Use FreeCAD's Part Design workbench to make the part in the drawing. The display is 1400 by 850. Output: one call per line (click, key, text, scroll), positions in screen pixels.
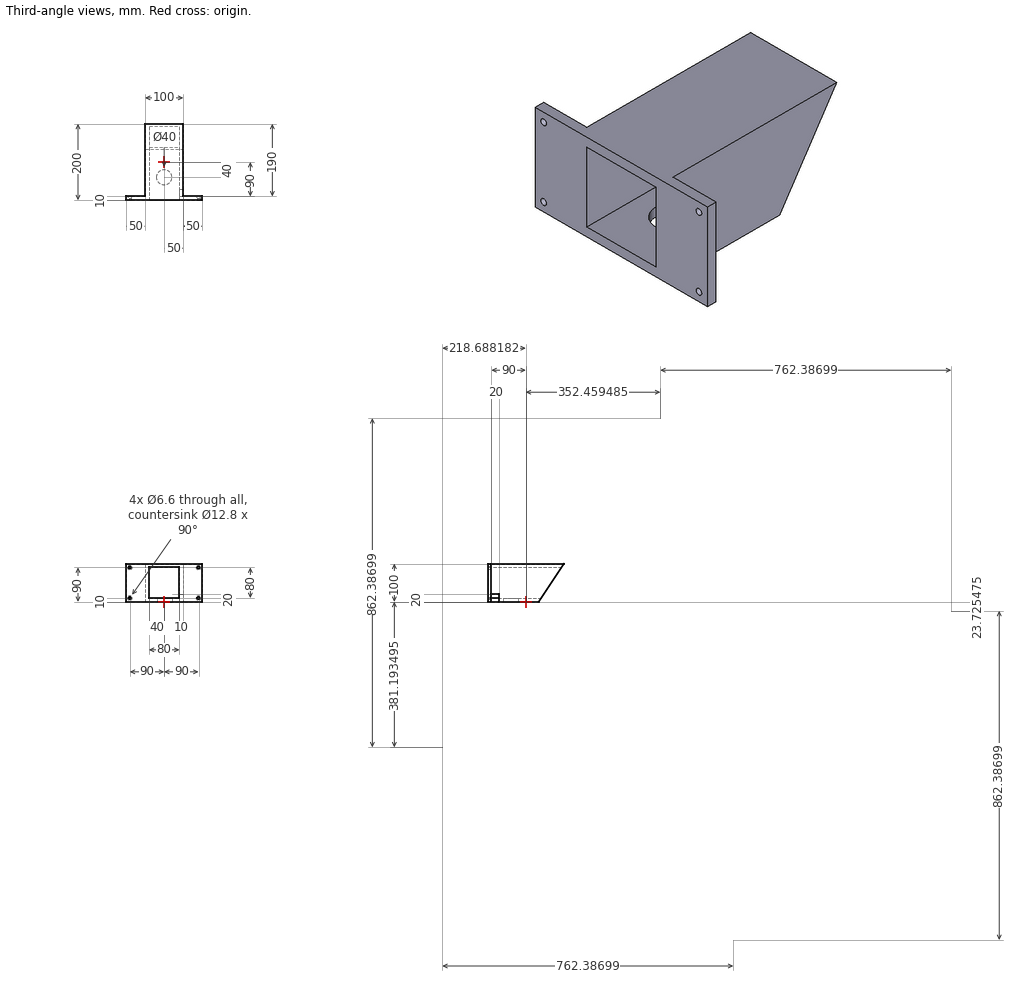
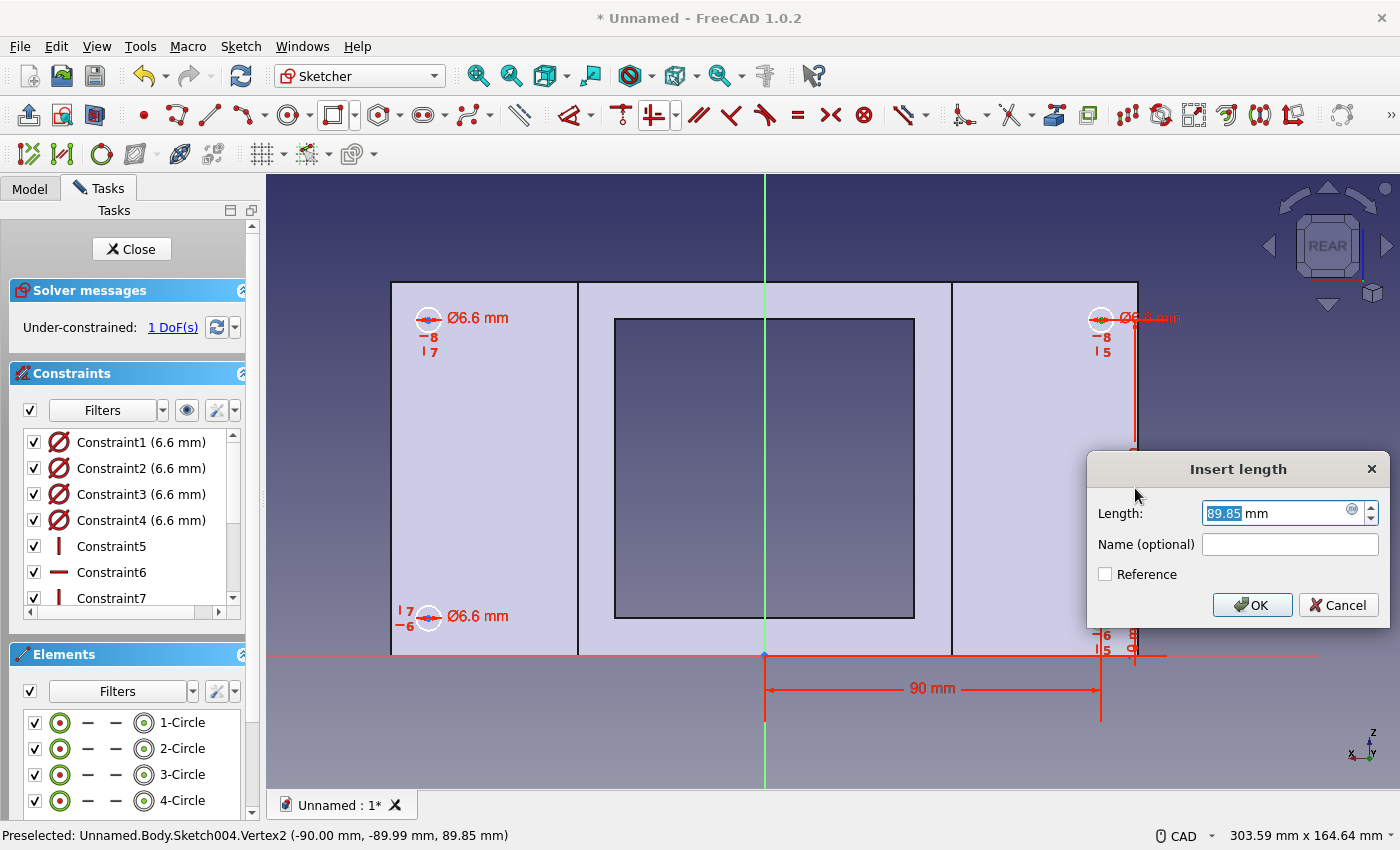
text(90)
key(Return)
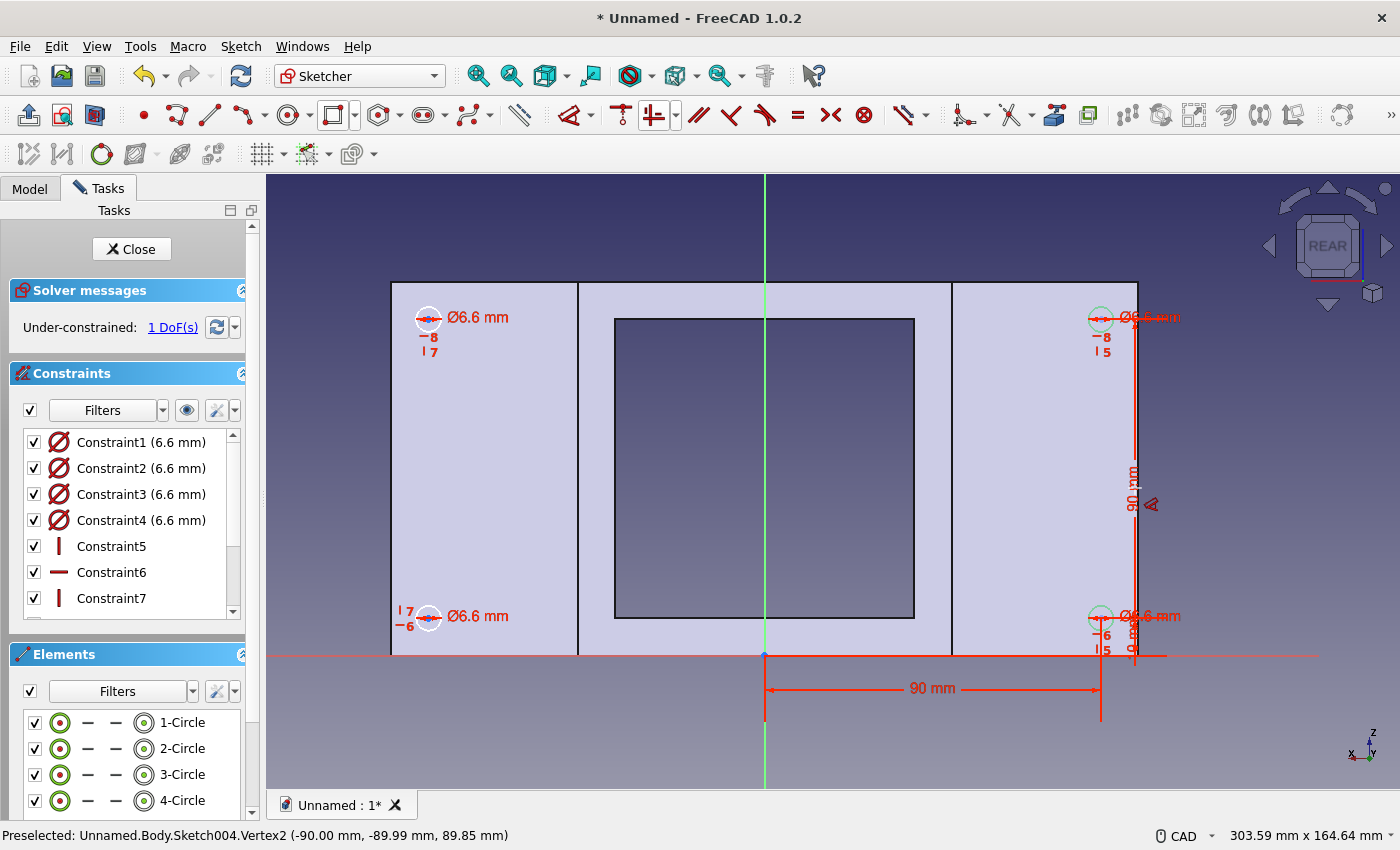
click(429, 618)
click(597, 690)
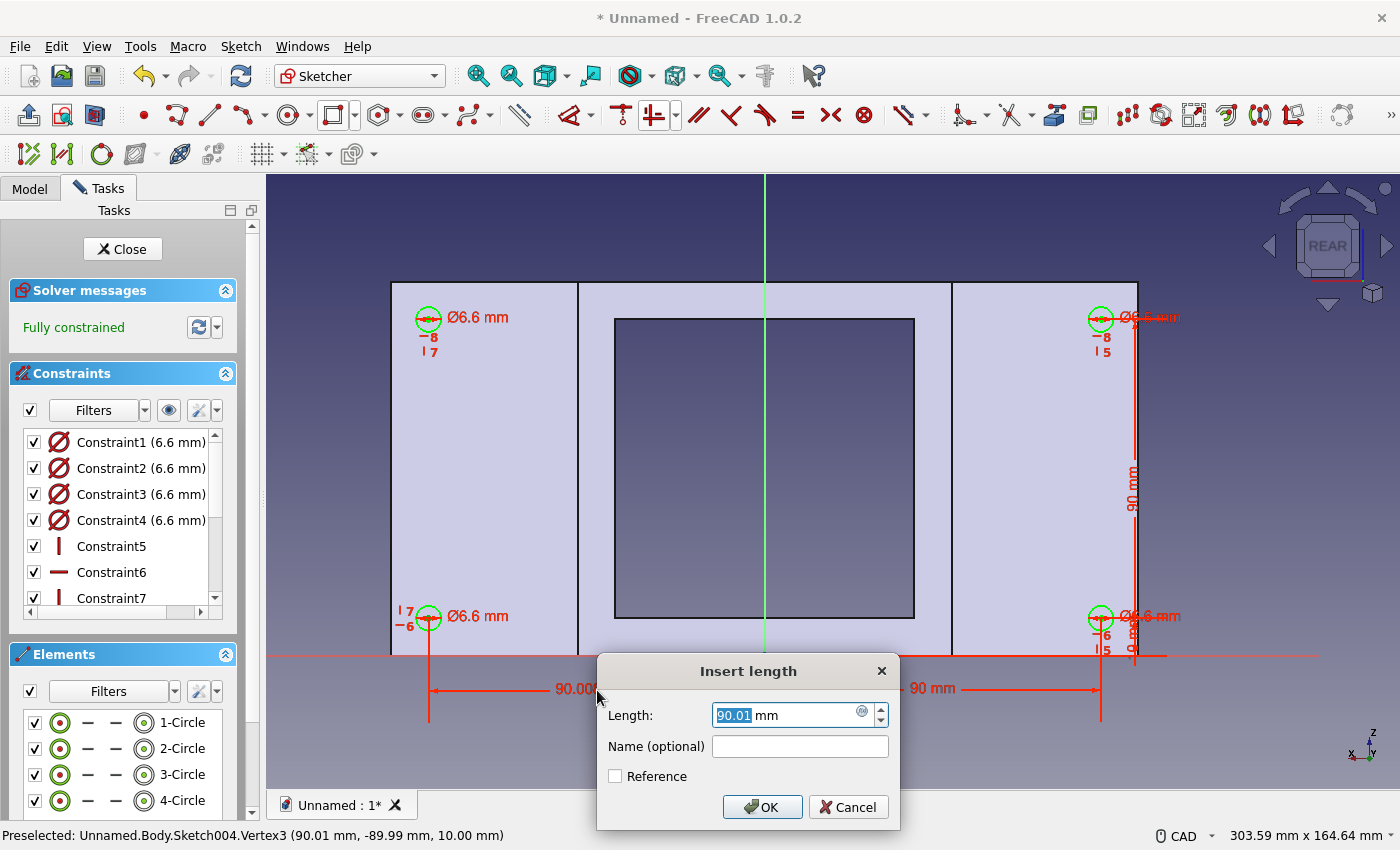
text(90)
key(Return)
key(Escape)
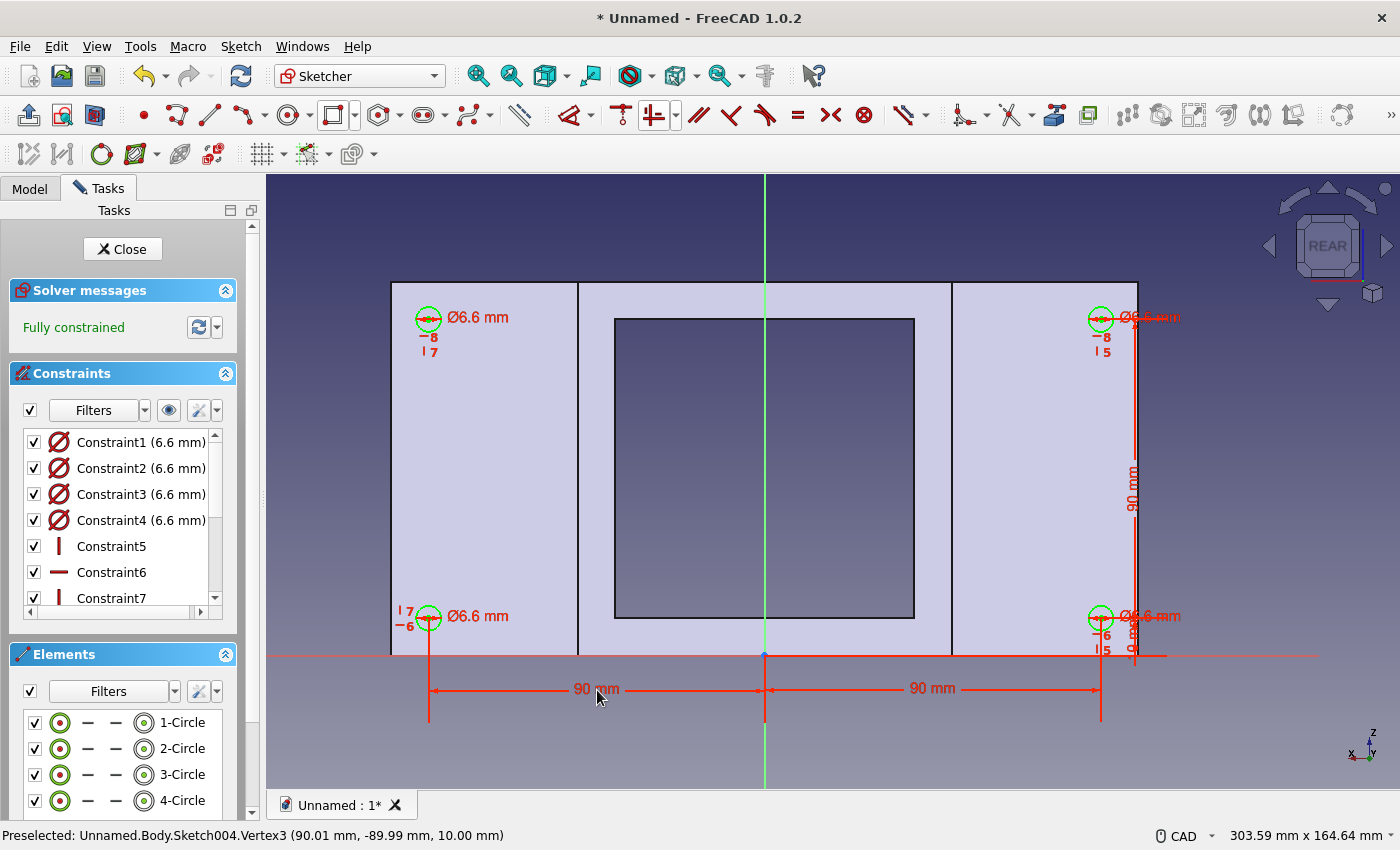
click(123, 249)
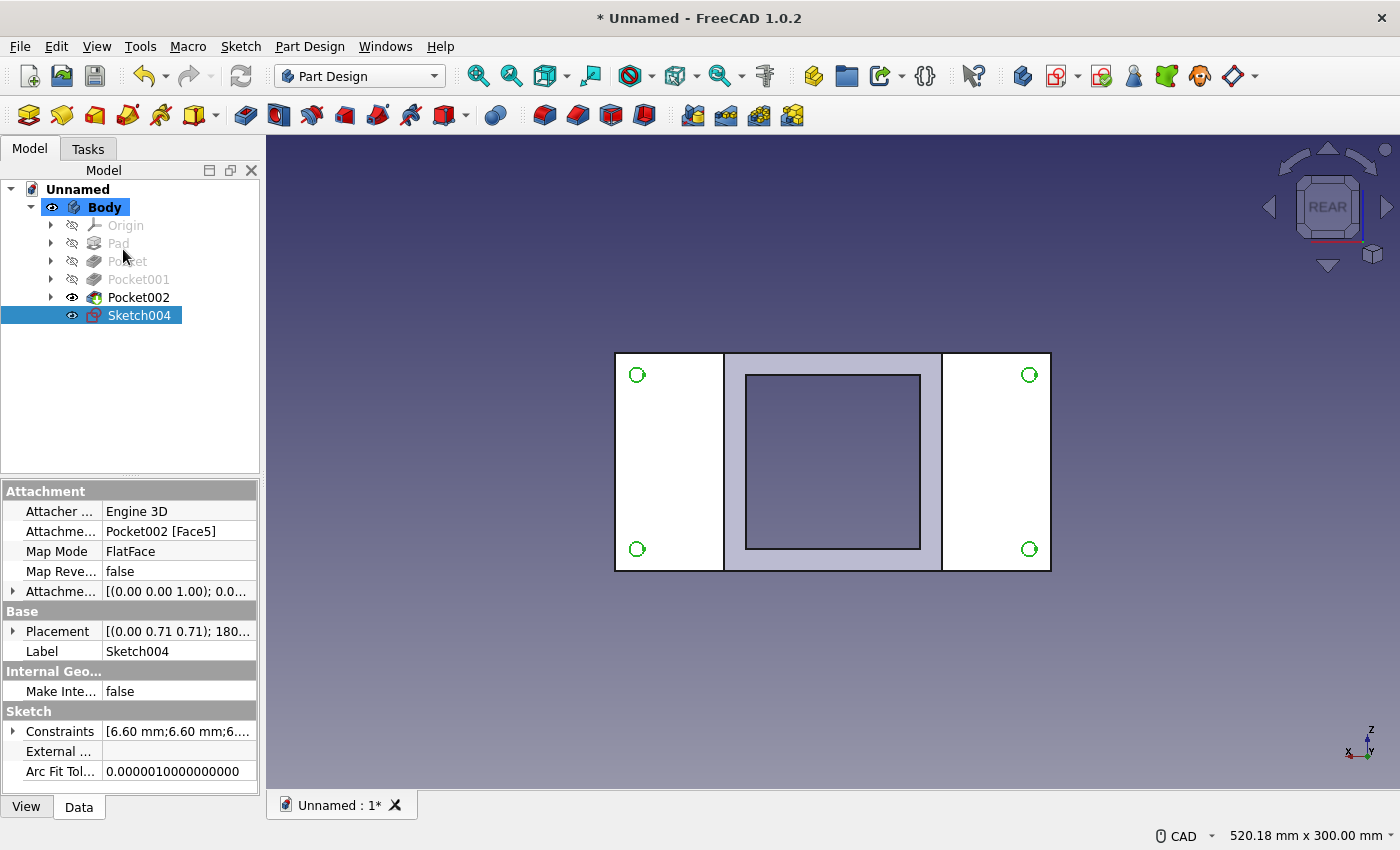
click(279, 116)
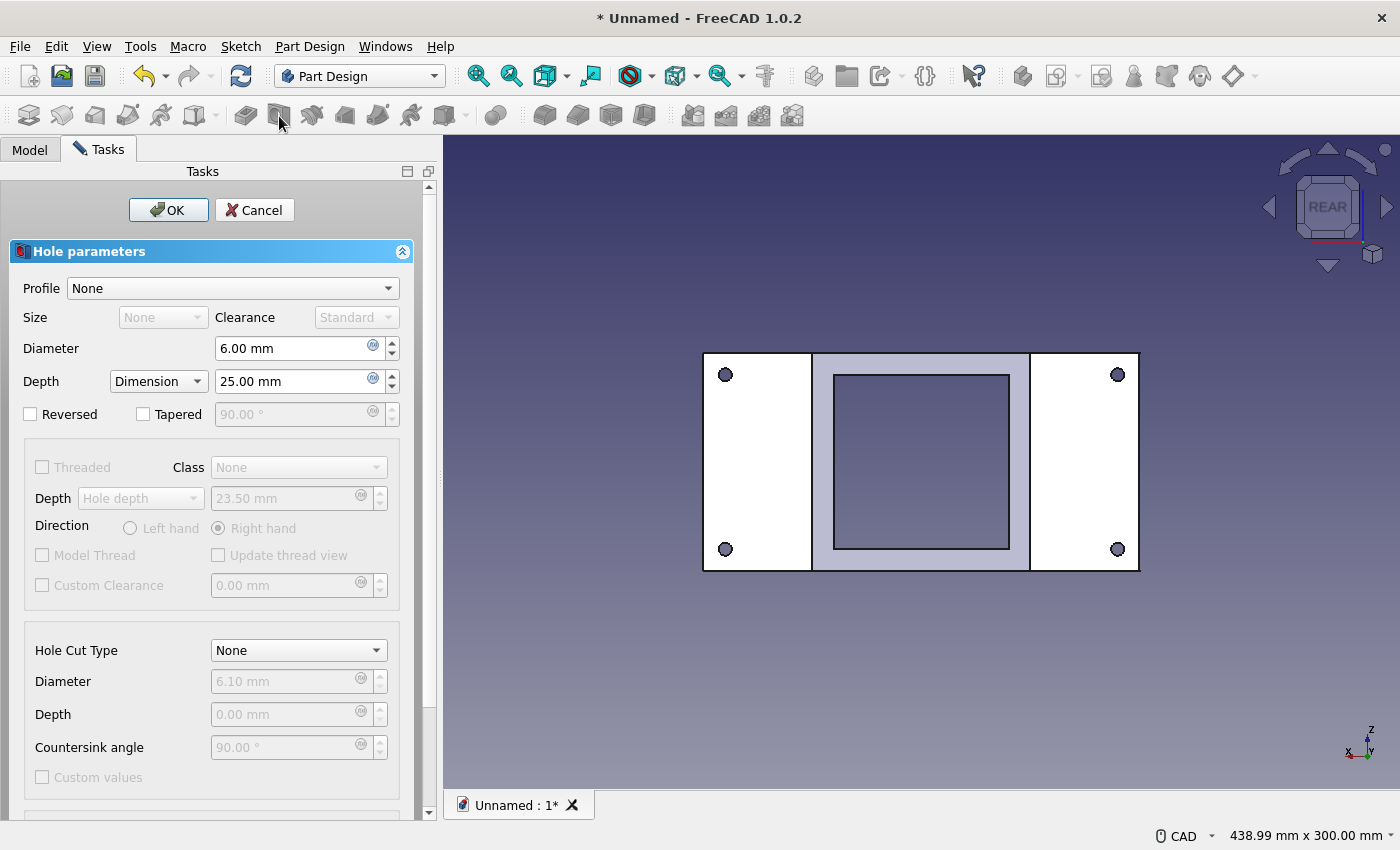
triple_click(300, 348)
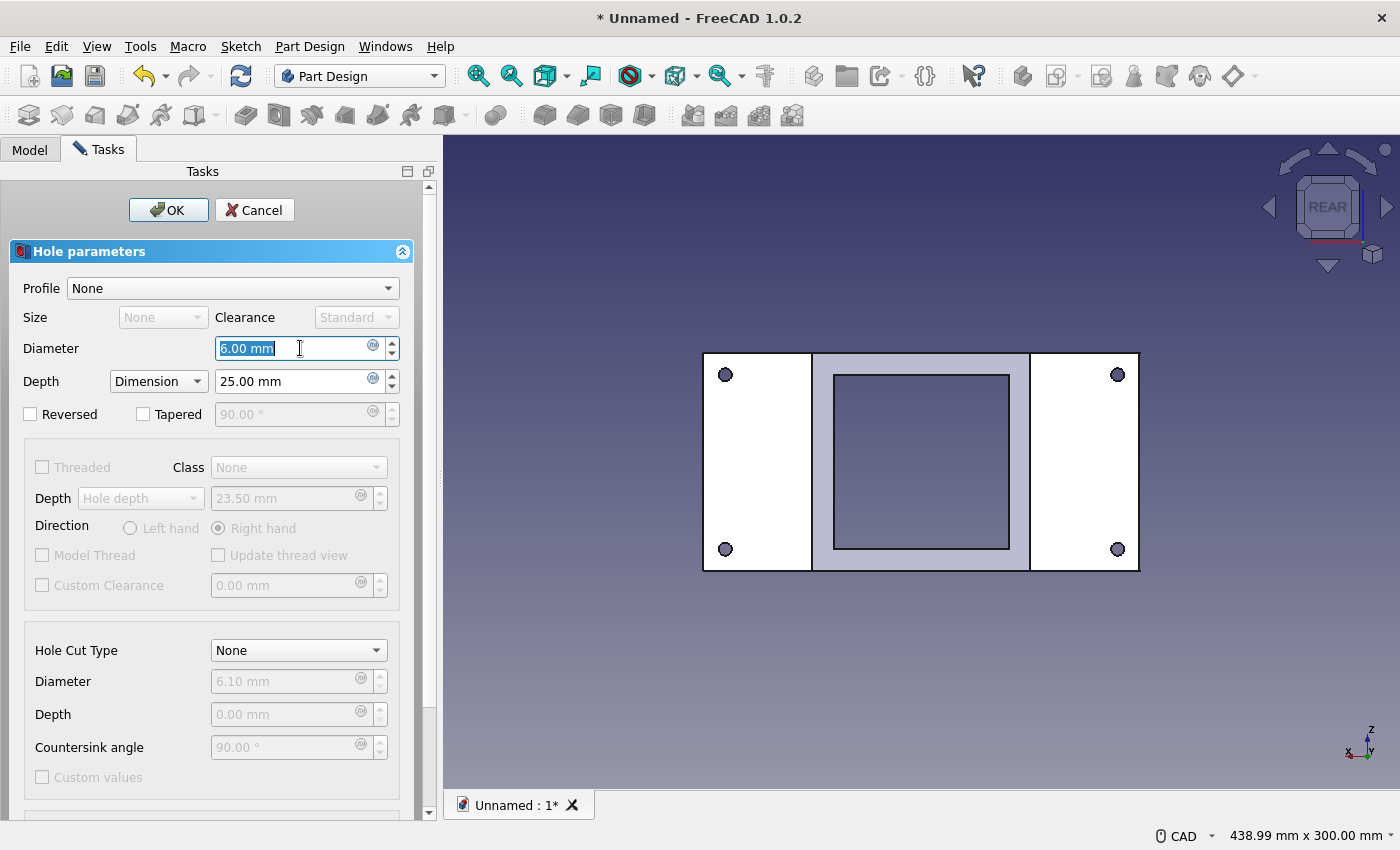
text(6.6)
key(Tab)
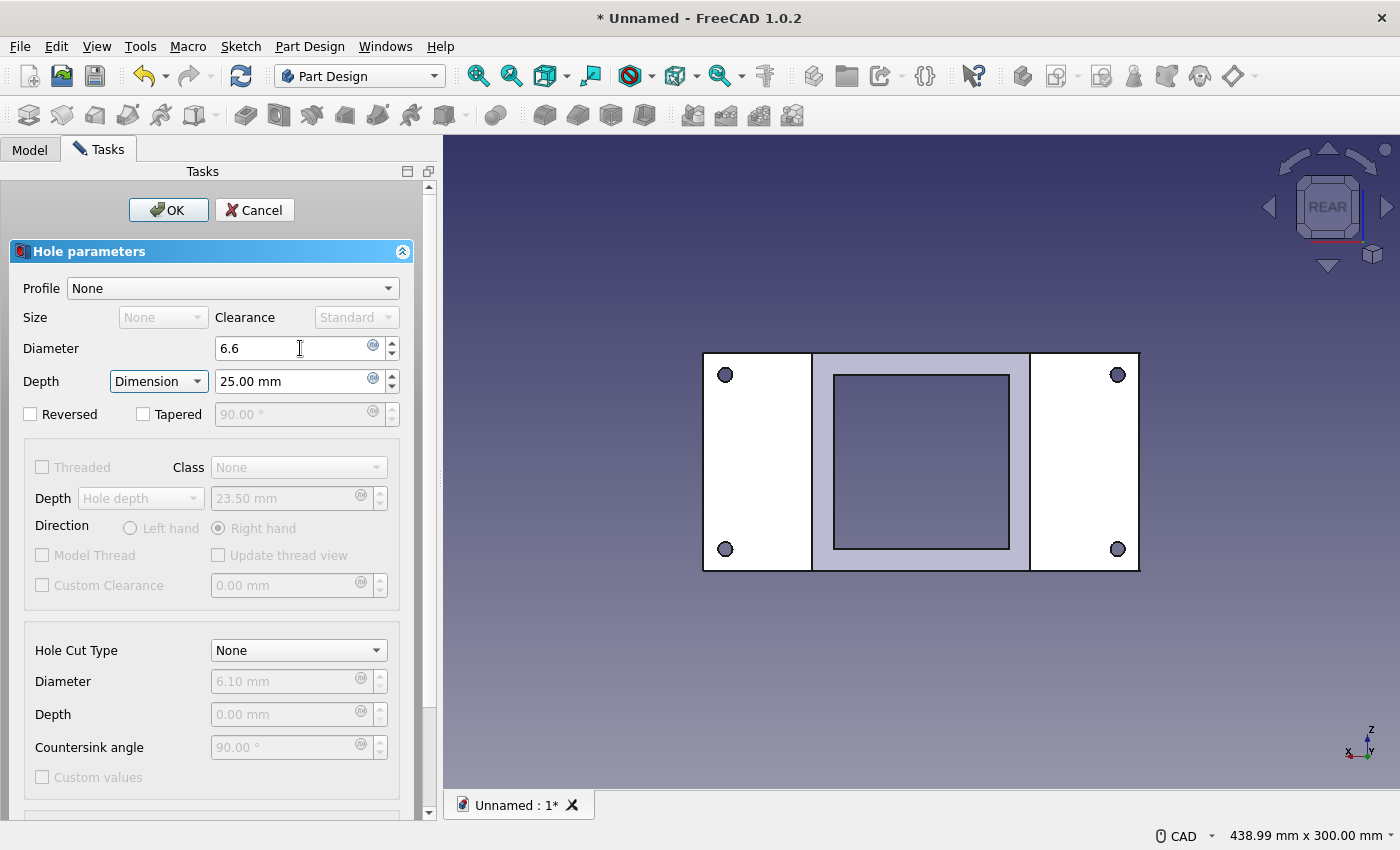
click(160, 382)